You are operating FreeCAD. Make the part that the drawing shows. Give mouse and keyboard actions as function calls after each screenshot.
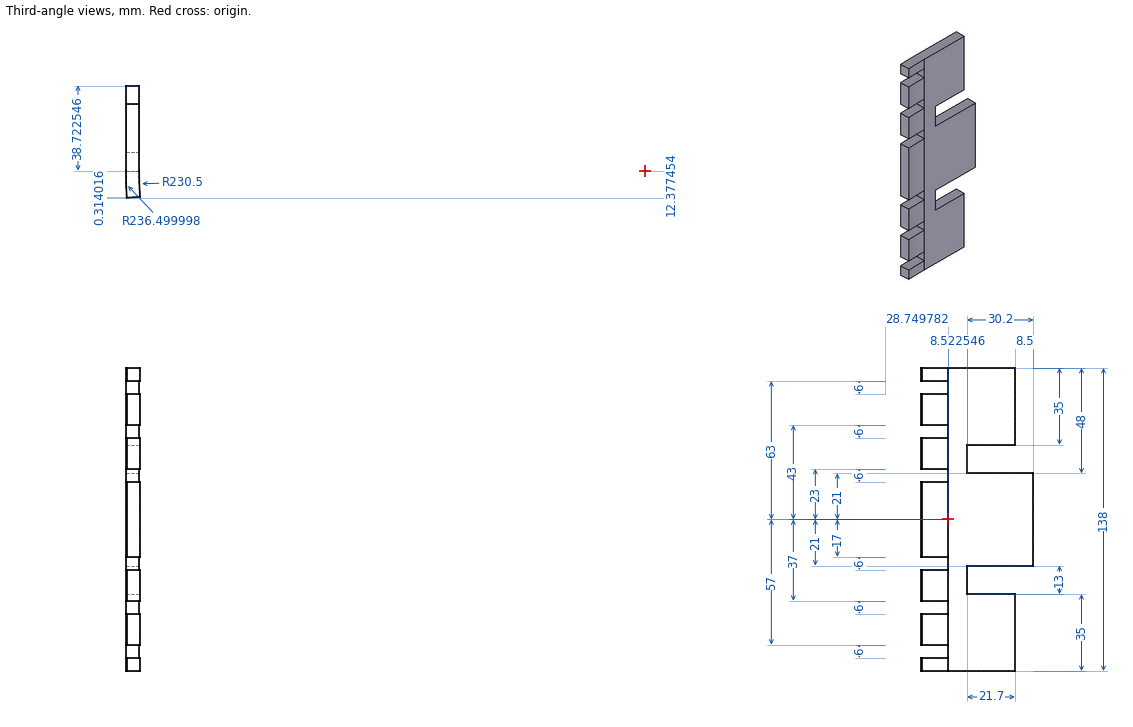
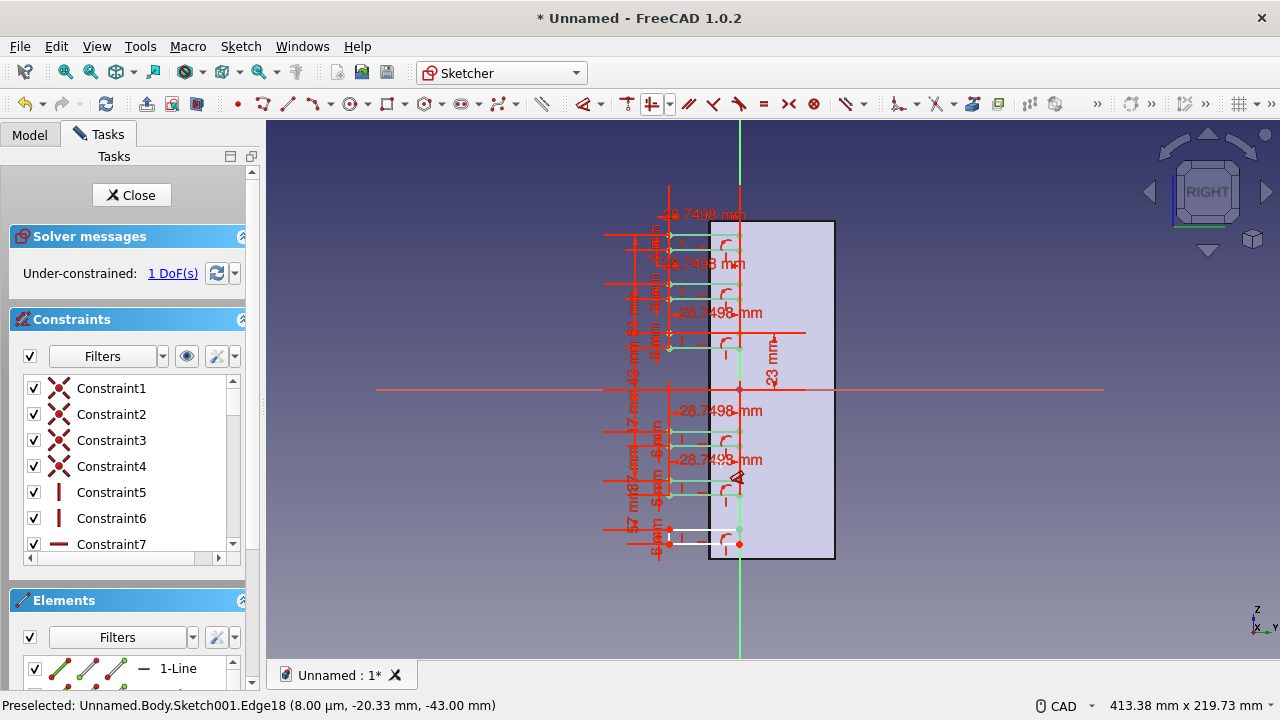
click(690, 544)
click(704, 578)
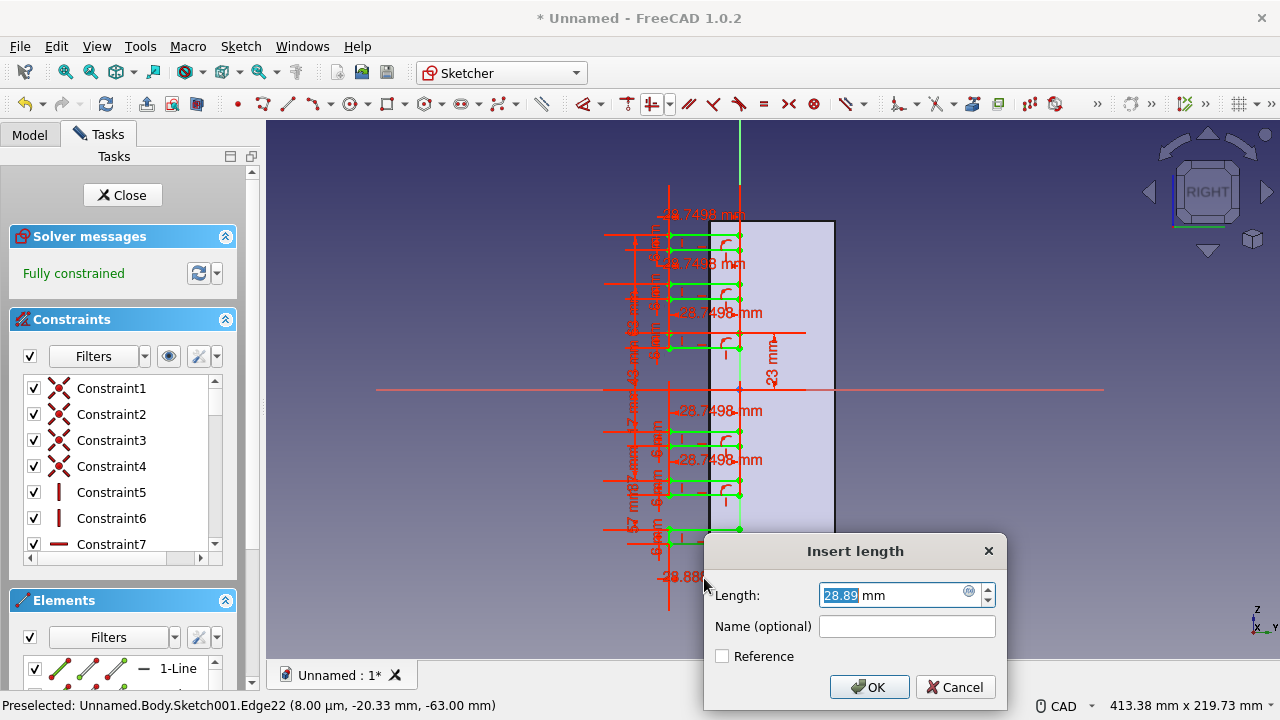
text(28.749782)
key(Return)
key(Escape)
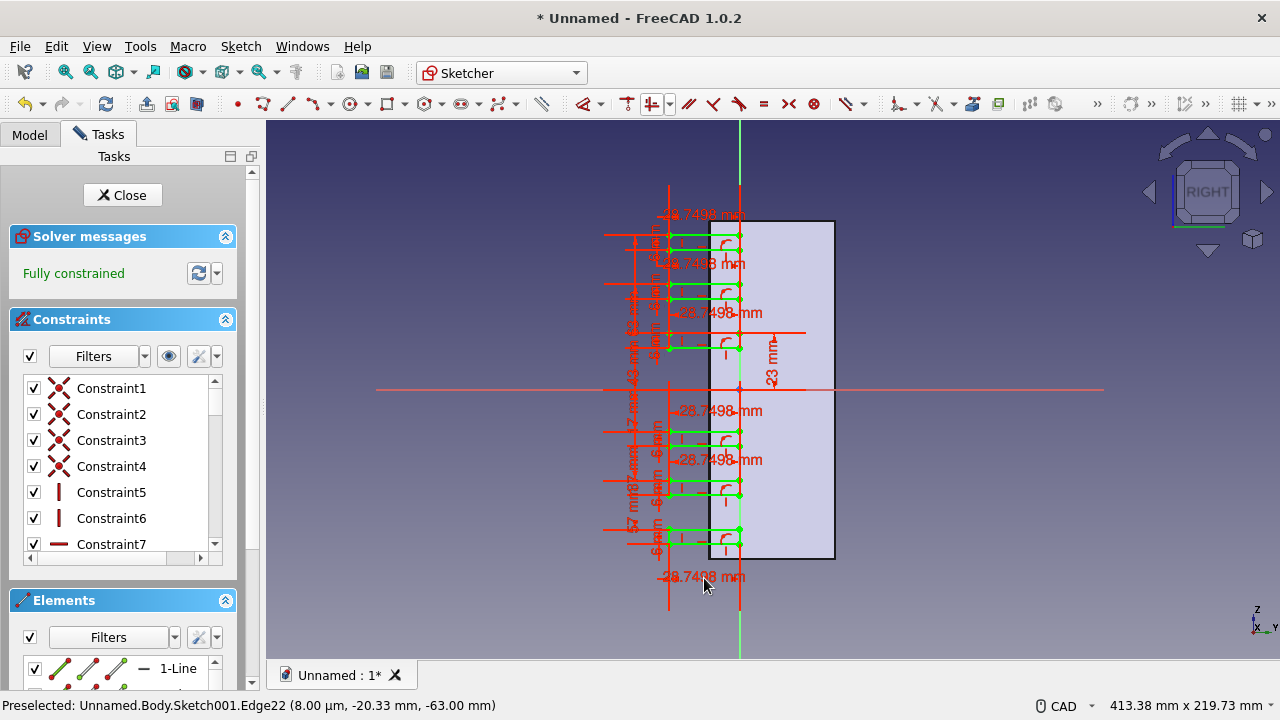
click(123, 195)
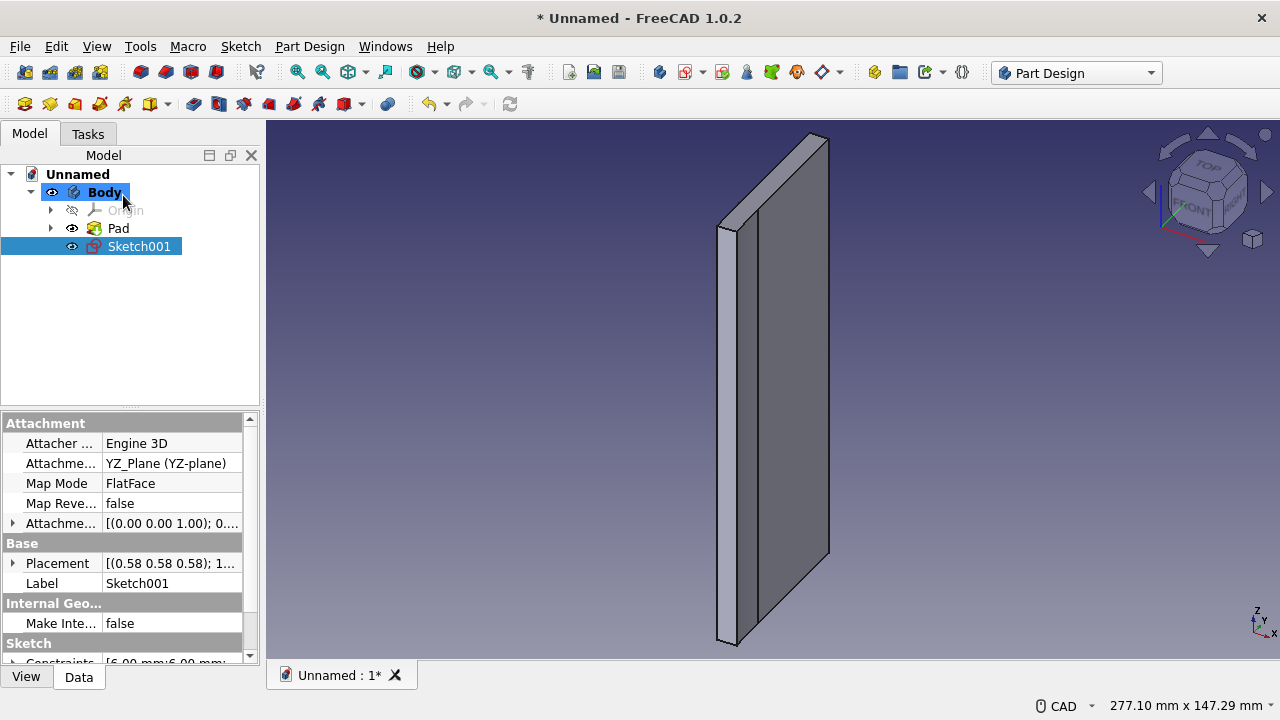
click(194, 104)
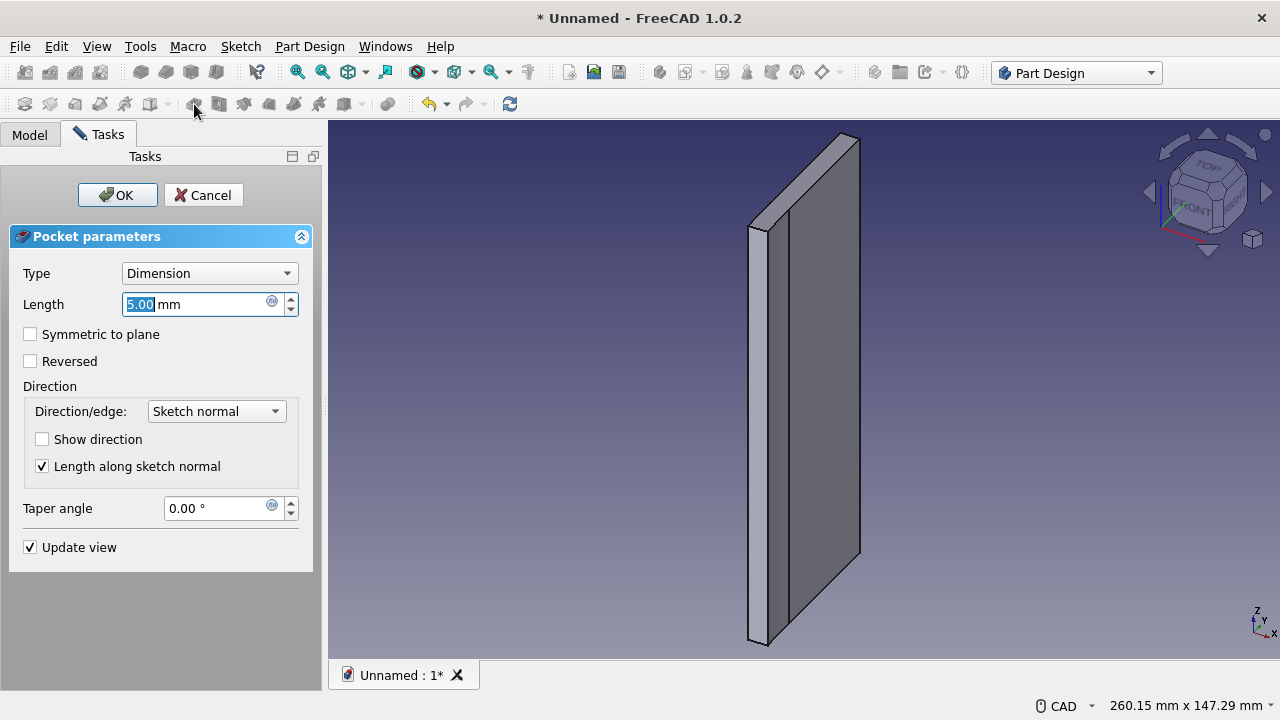
click(210, 274)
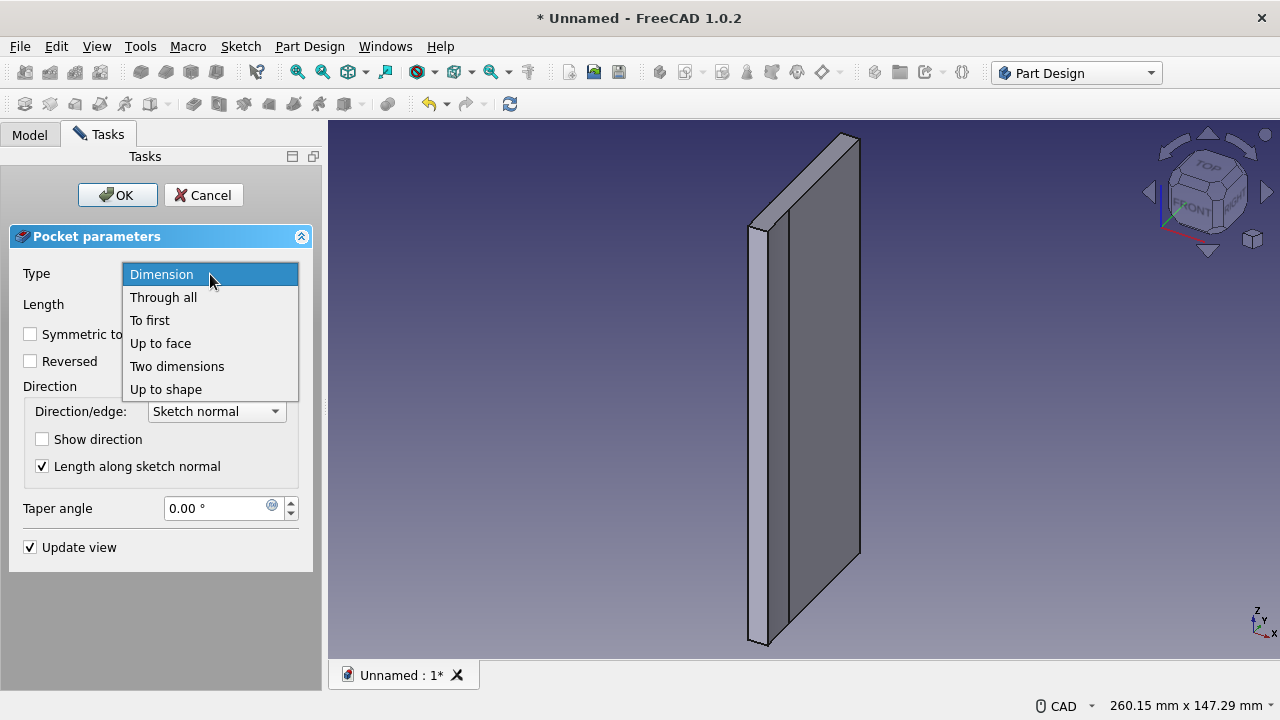
click(208, 298)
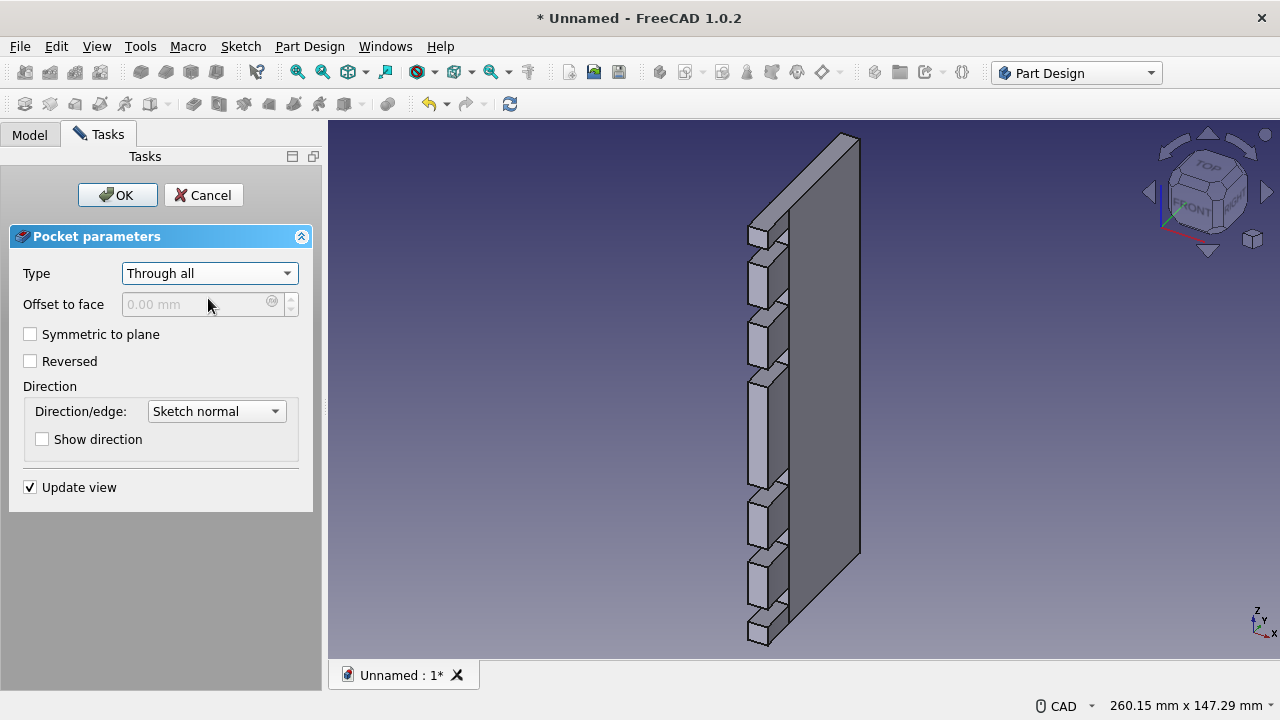
click(118, 195)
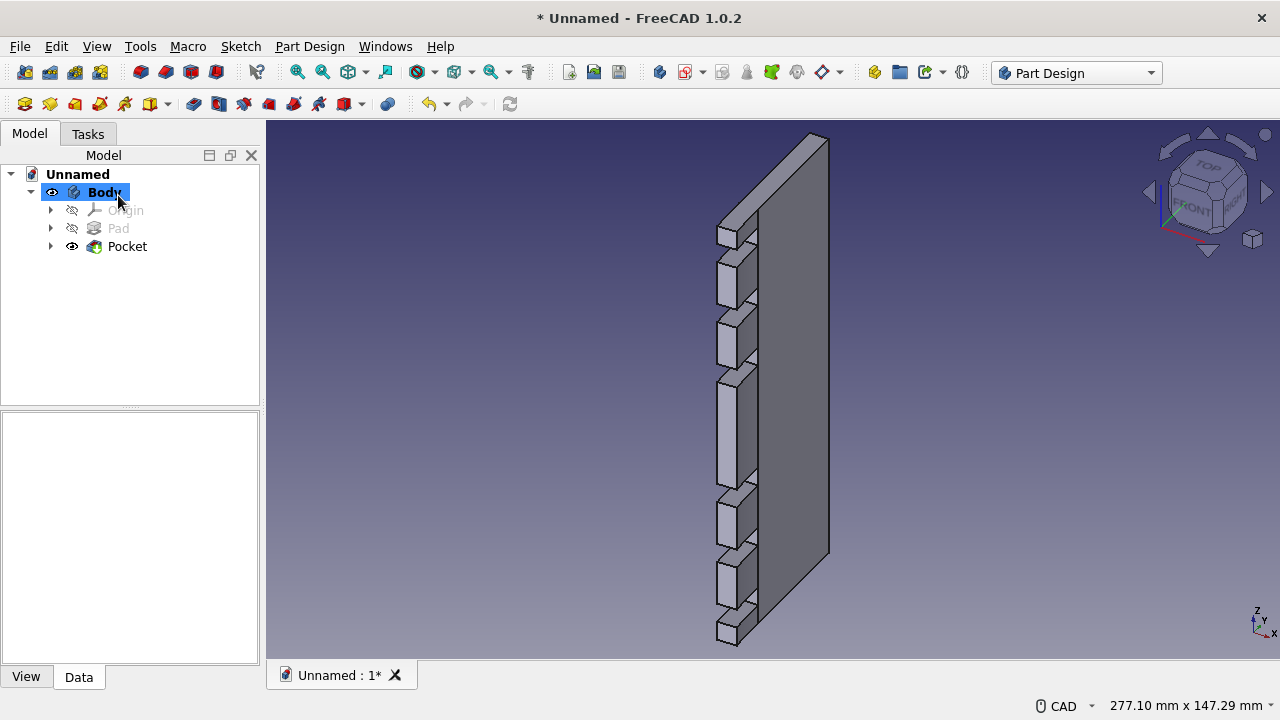
click(793, 262)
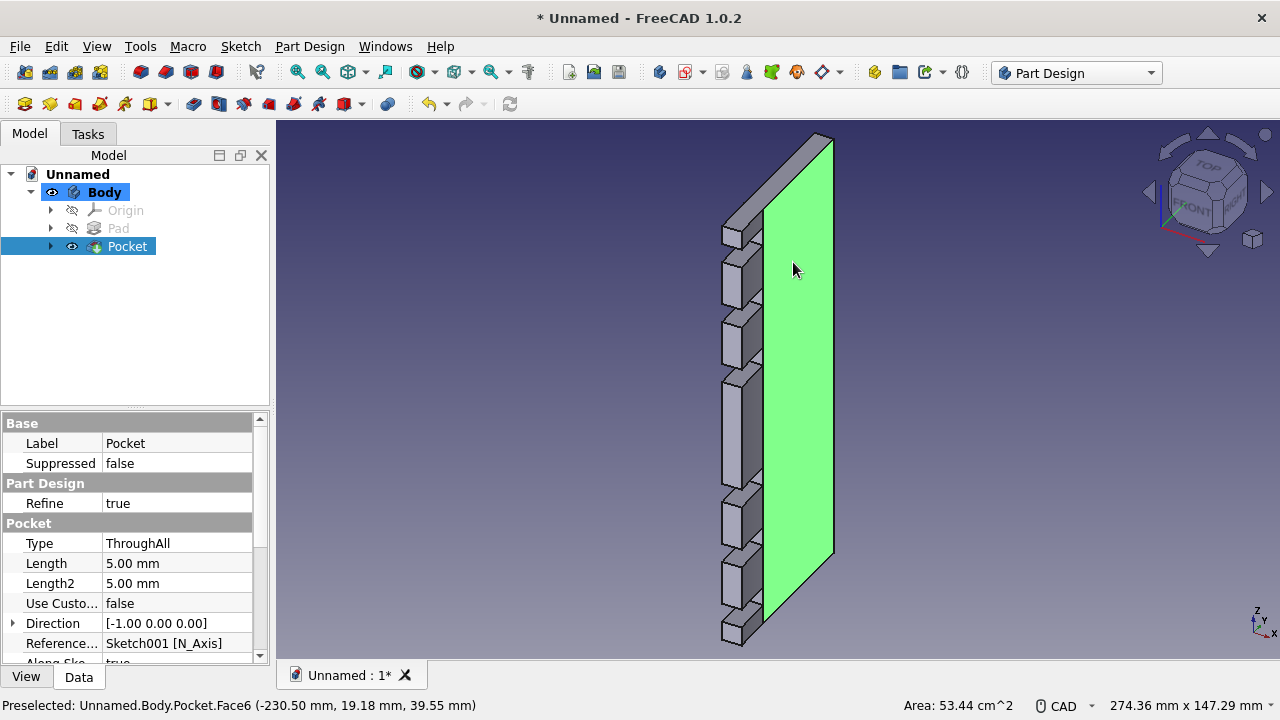
click(684, 72)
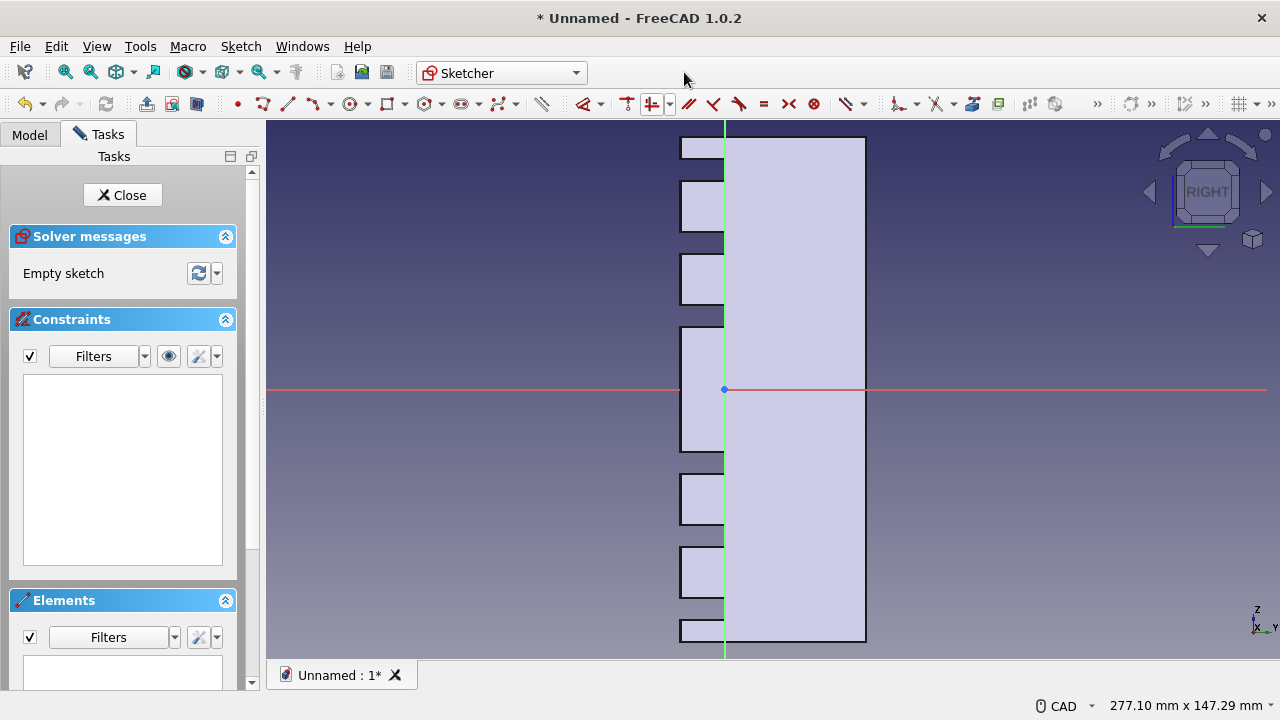
scroll(519, 390, down, 2)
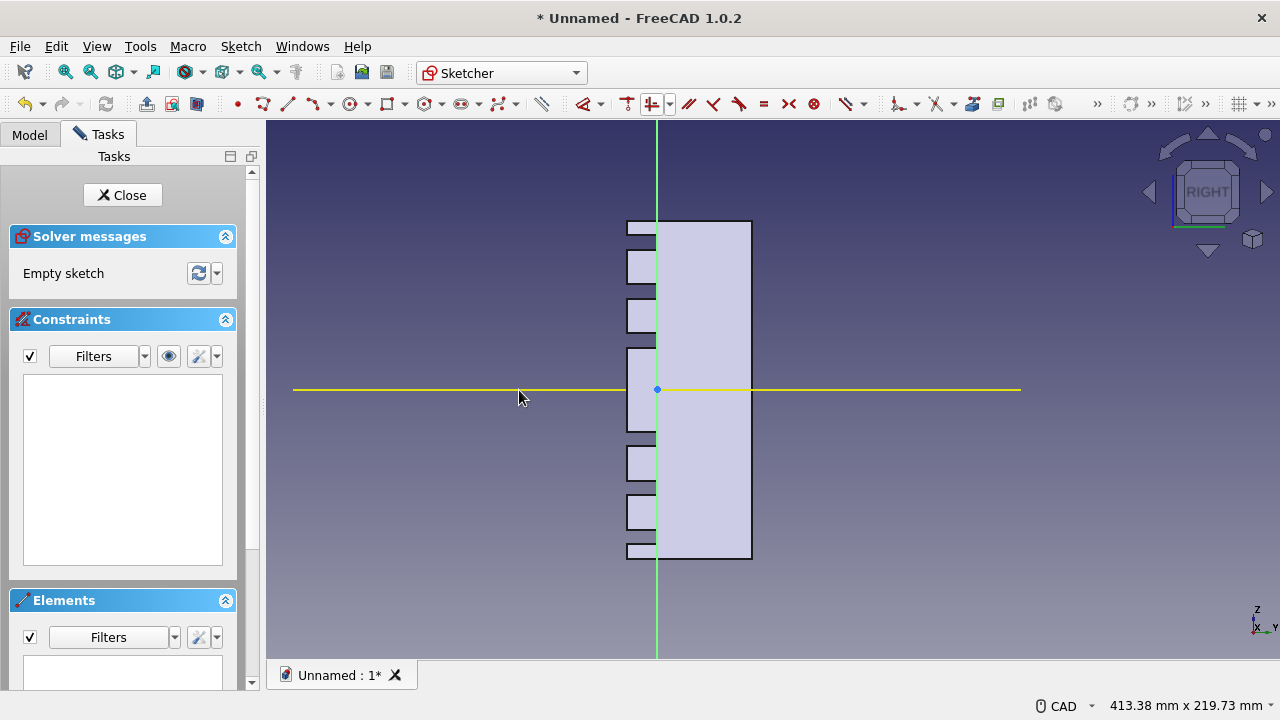
key(g)
key(m)